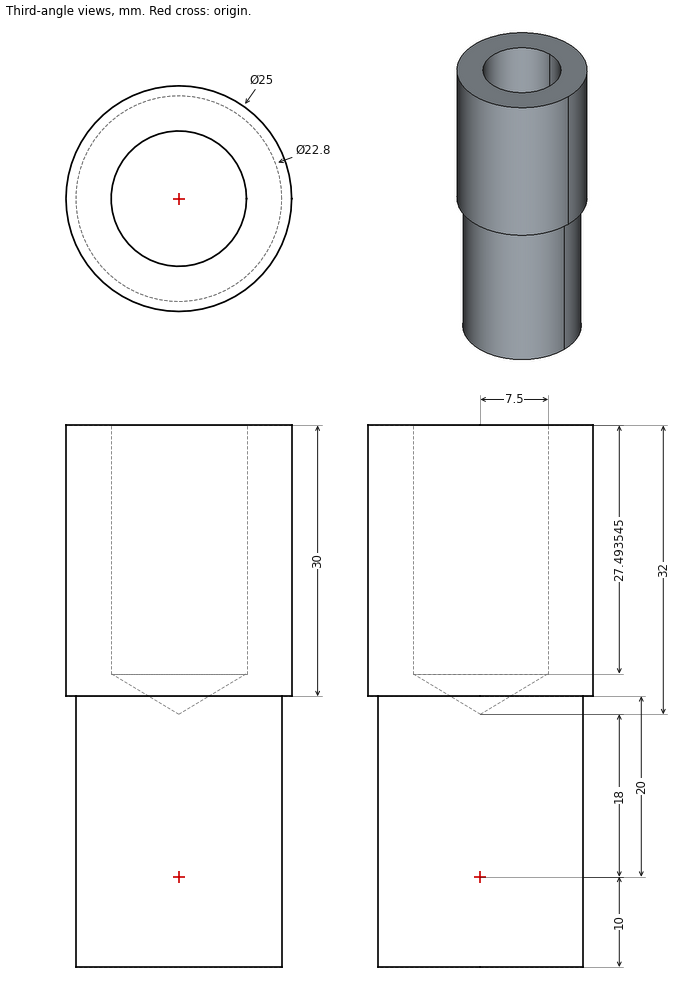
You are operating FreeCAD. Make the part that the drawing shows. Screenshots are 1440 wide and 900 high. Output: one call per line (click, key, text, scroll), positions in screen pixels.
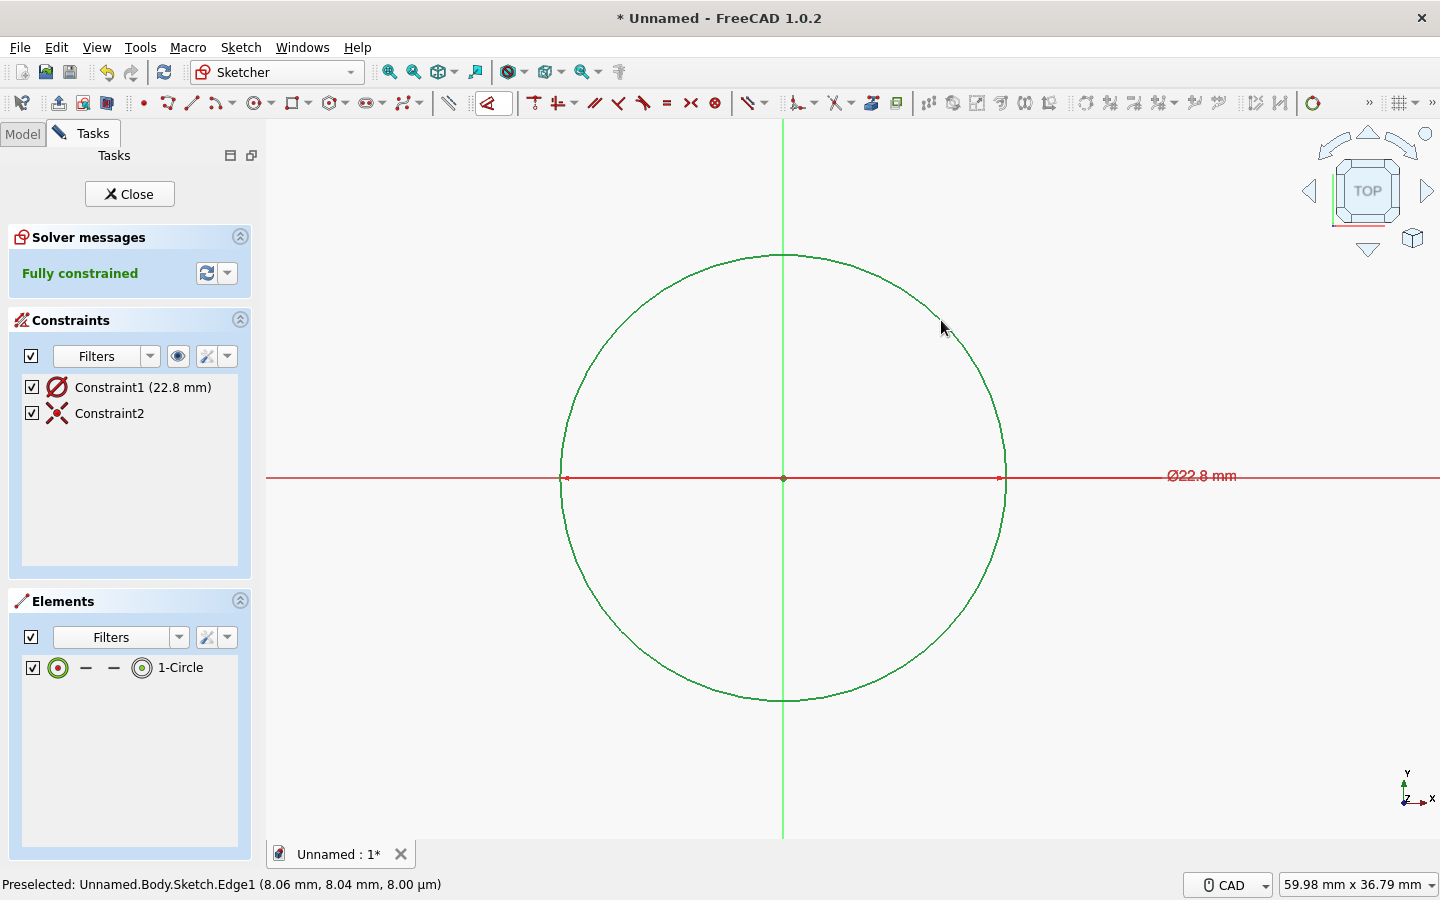
click(130, 194)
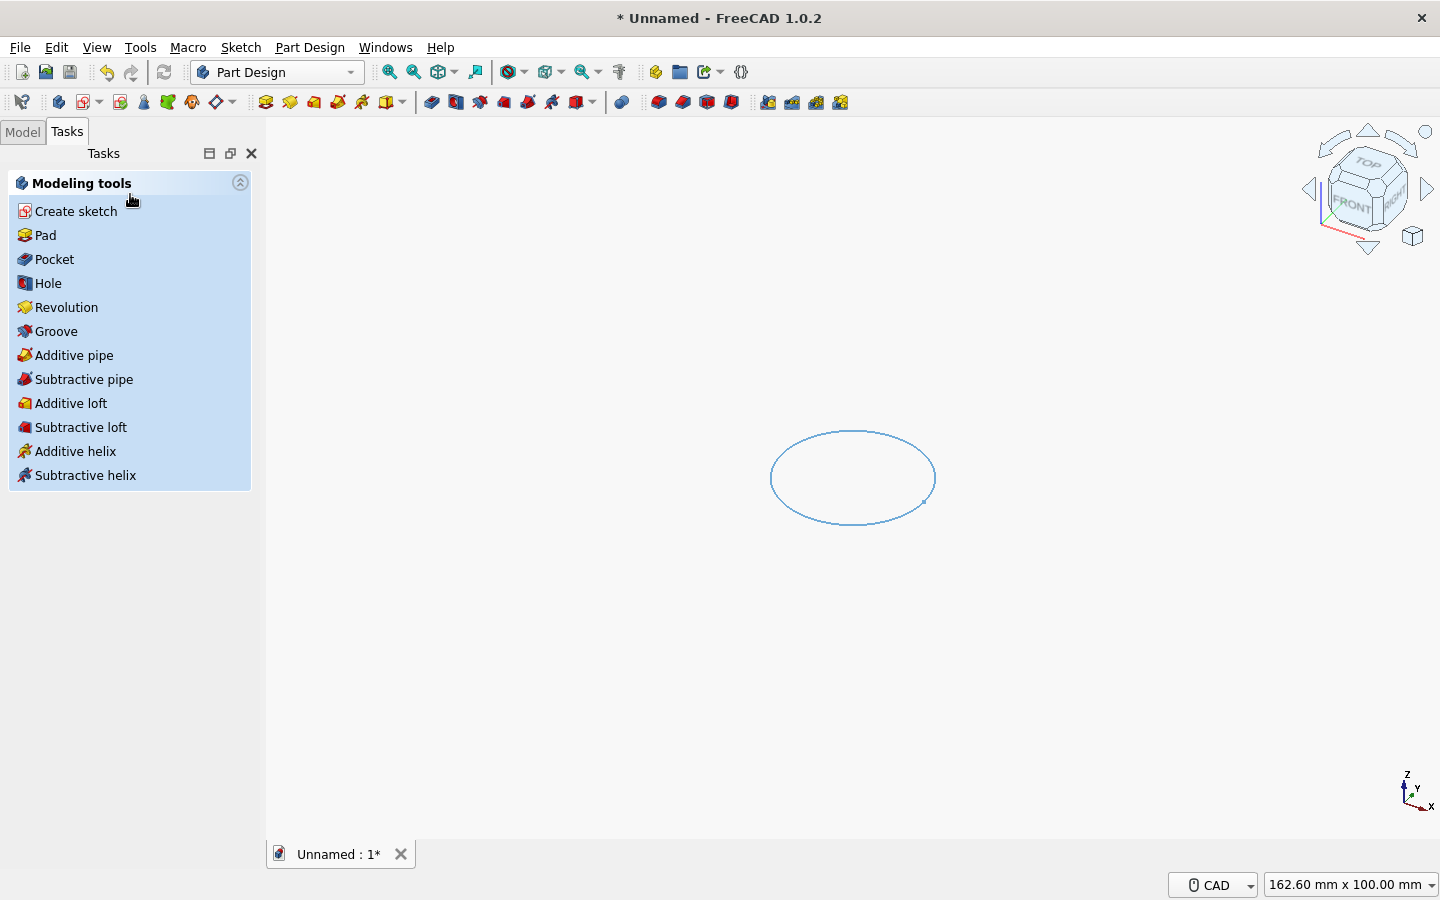
click(266, 102)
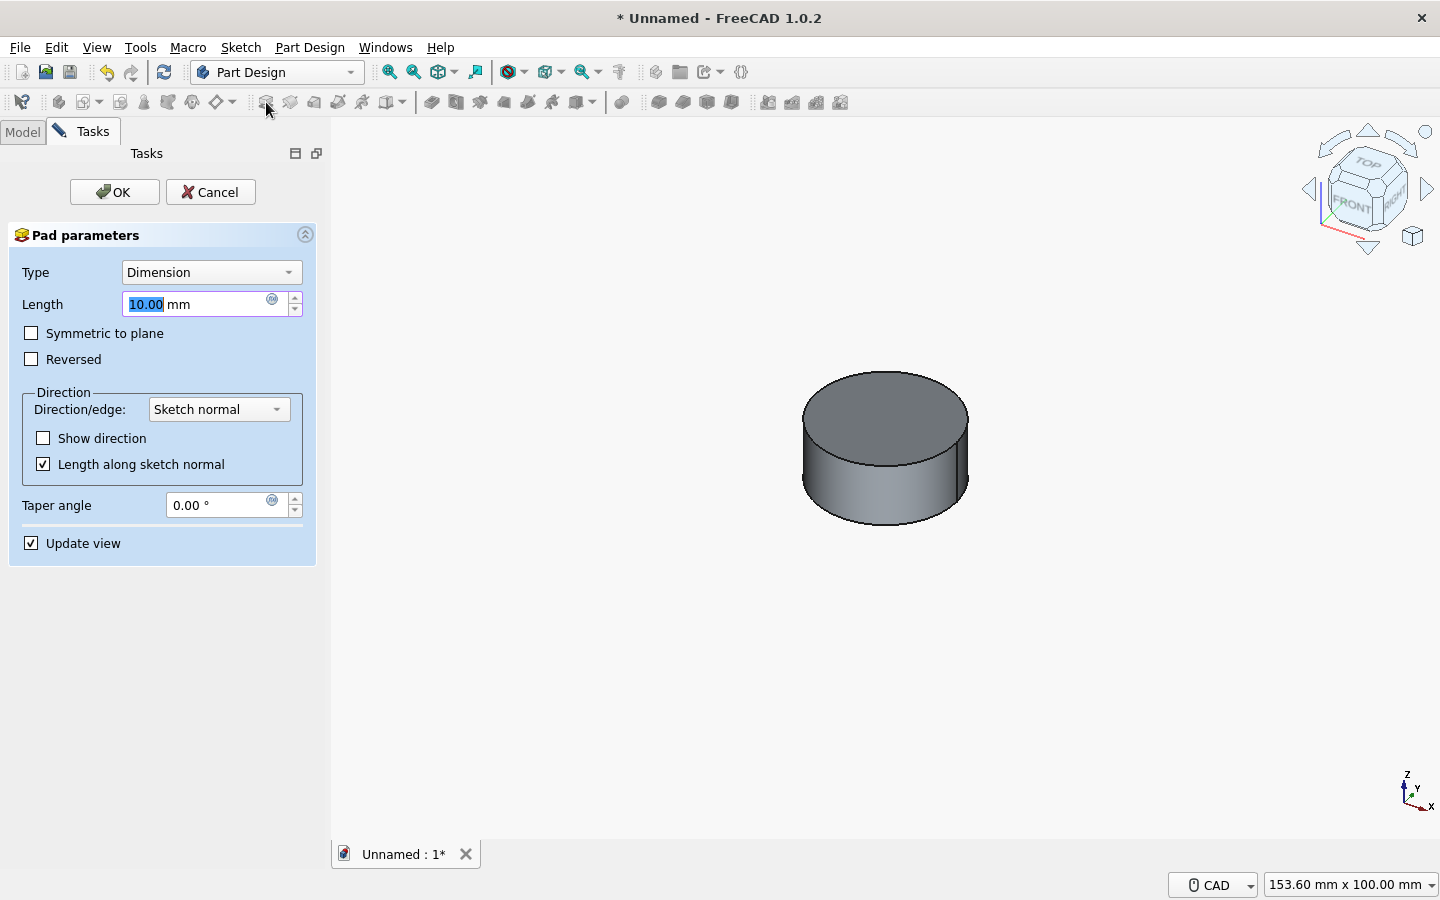
click(212, 272)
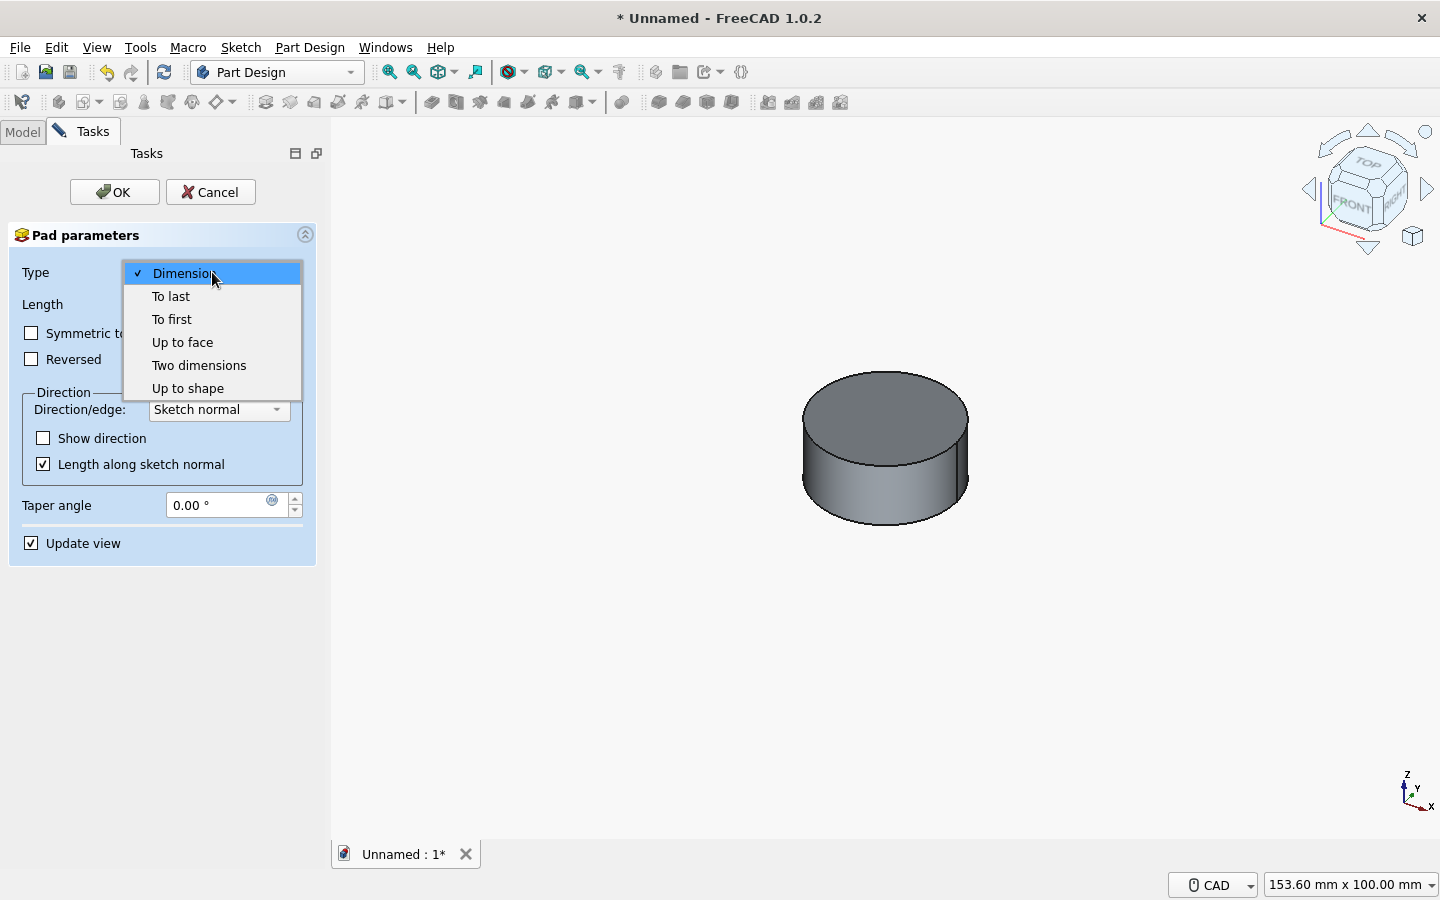
click(212, 366)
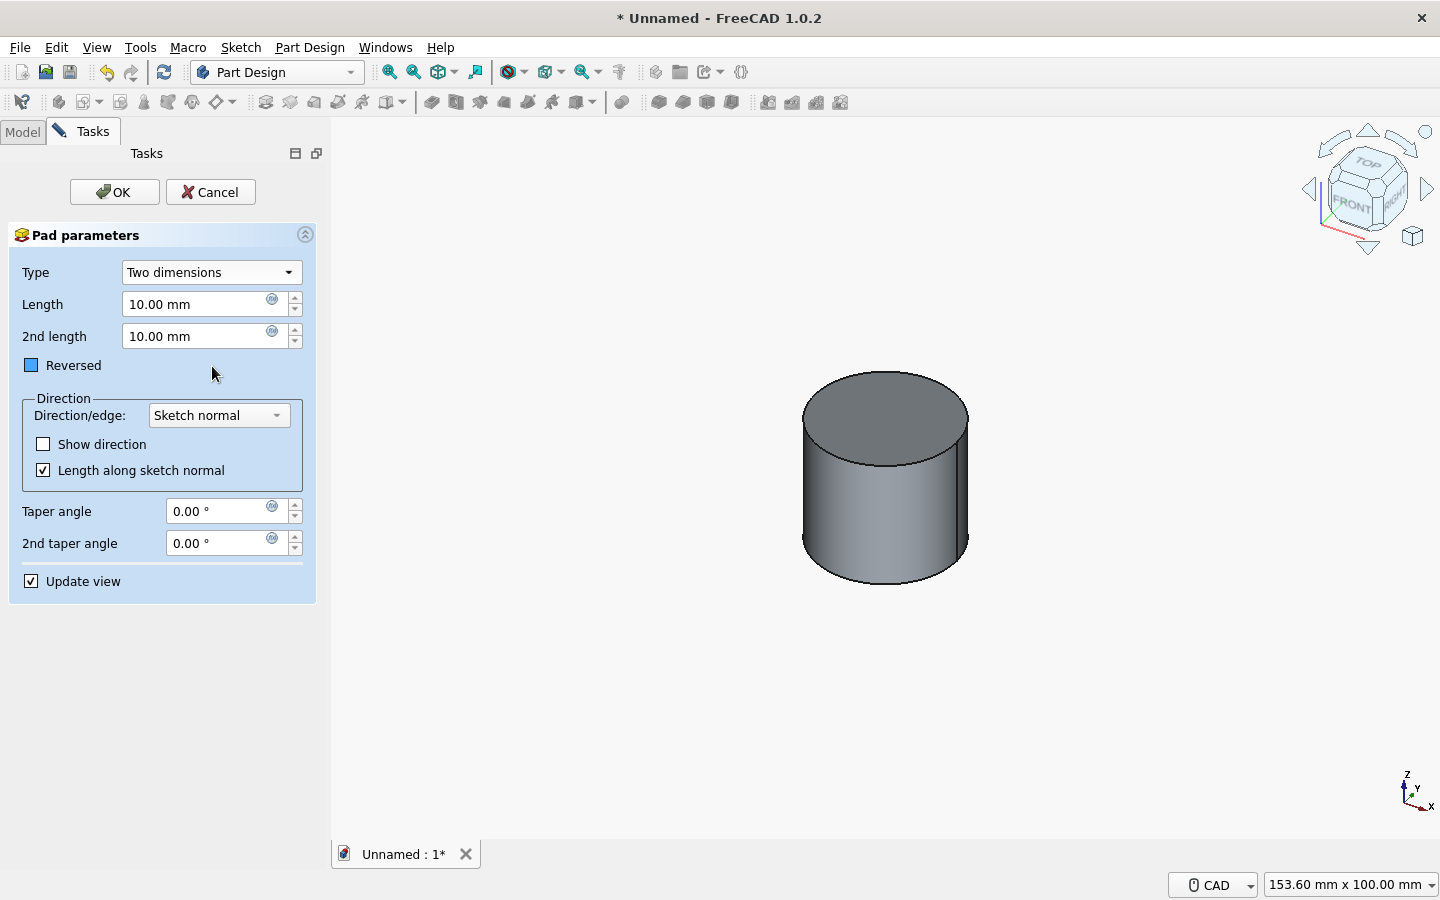
triple_click(204, 304)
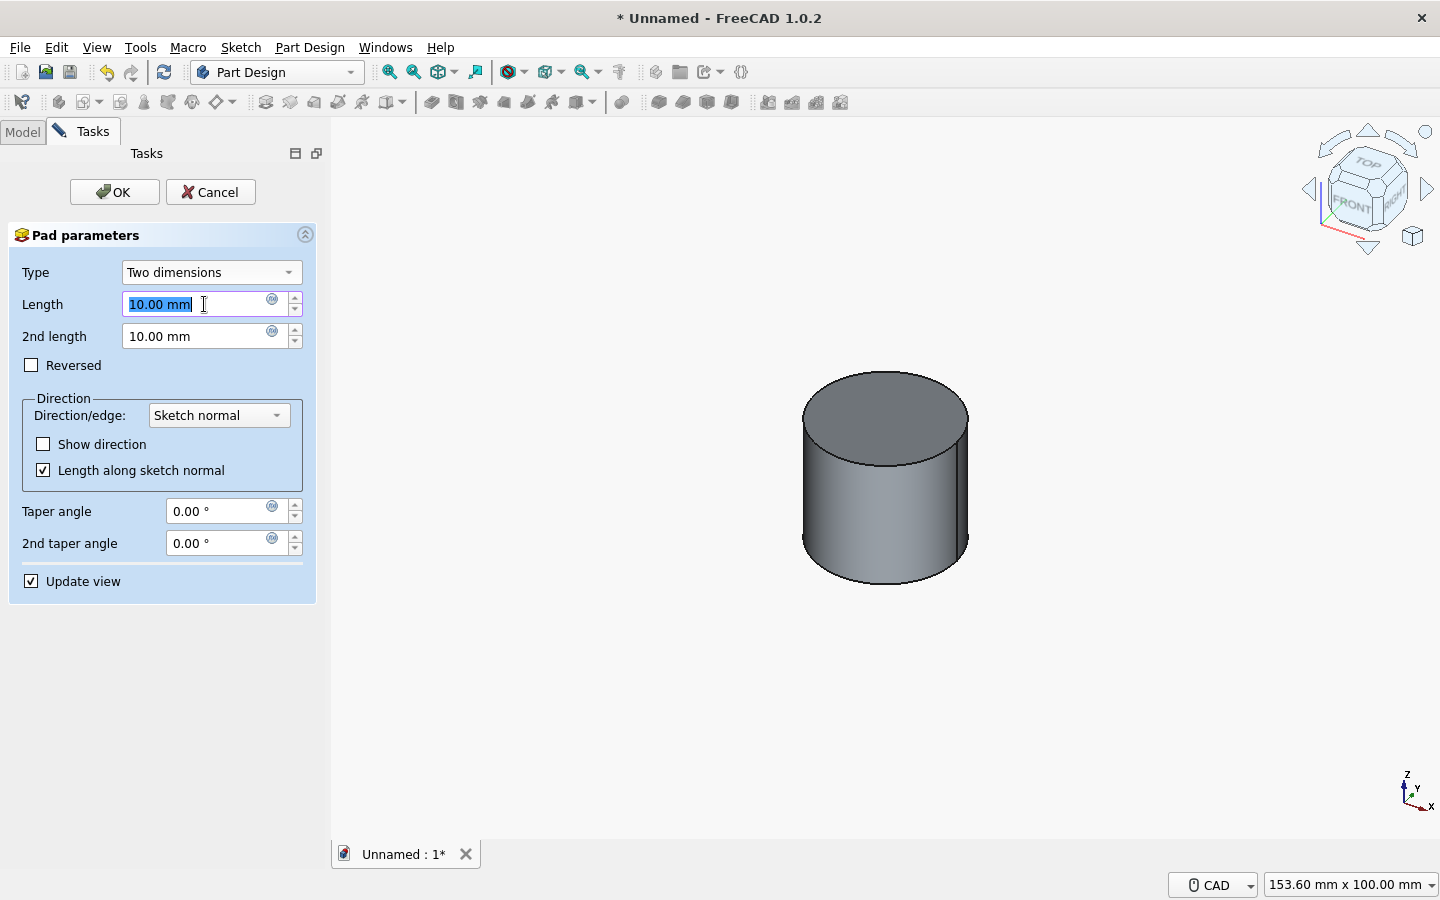
text(20)
key(Tab)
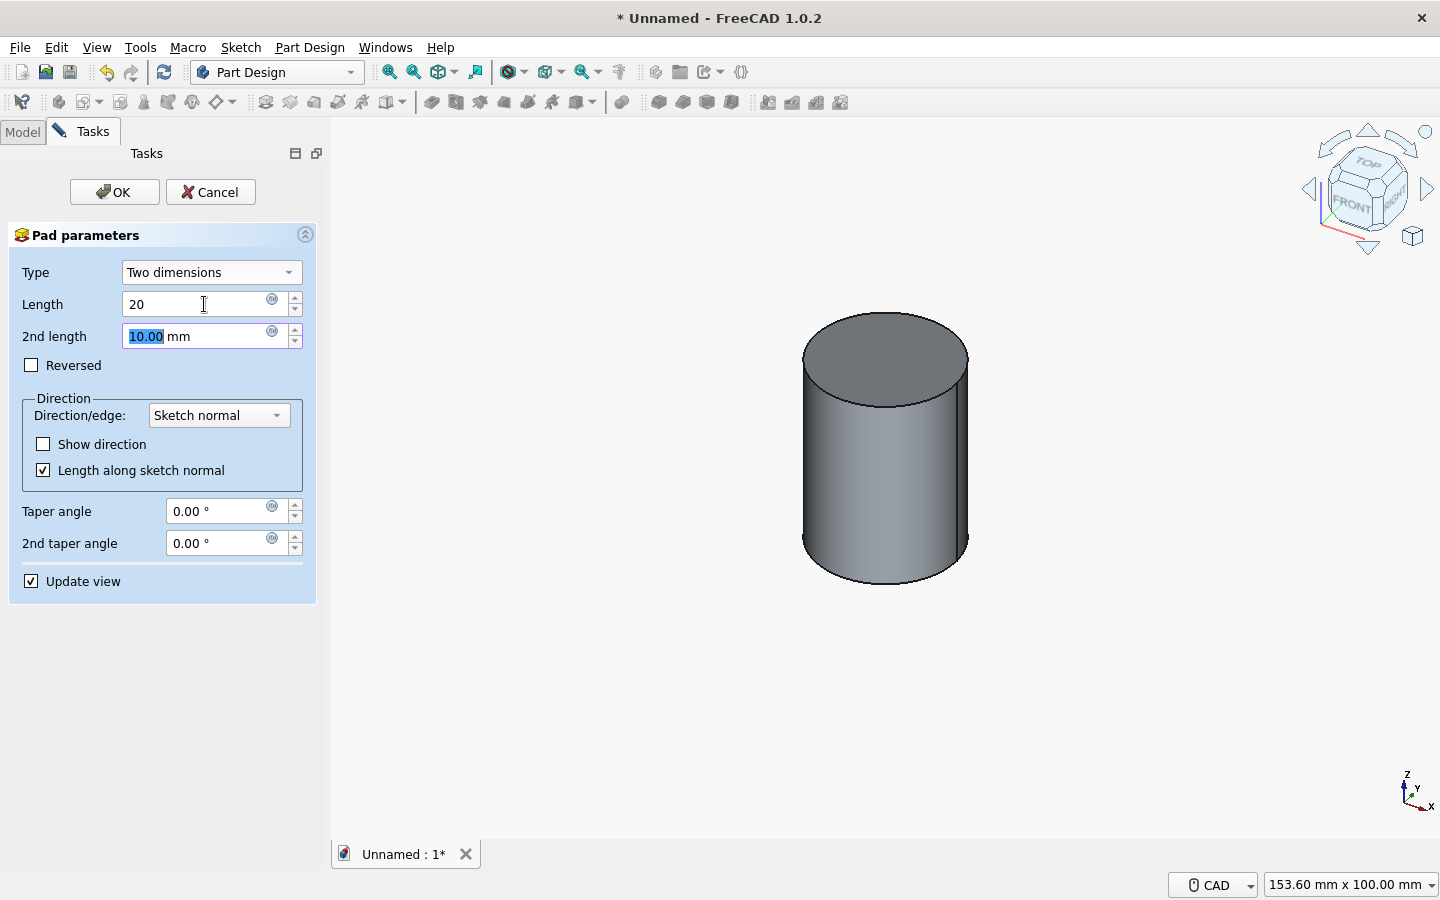
text(10)
key(Tab)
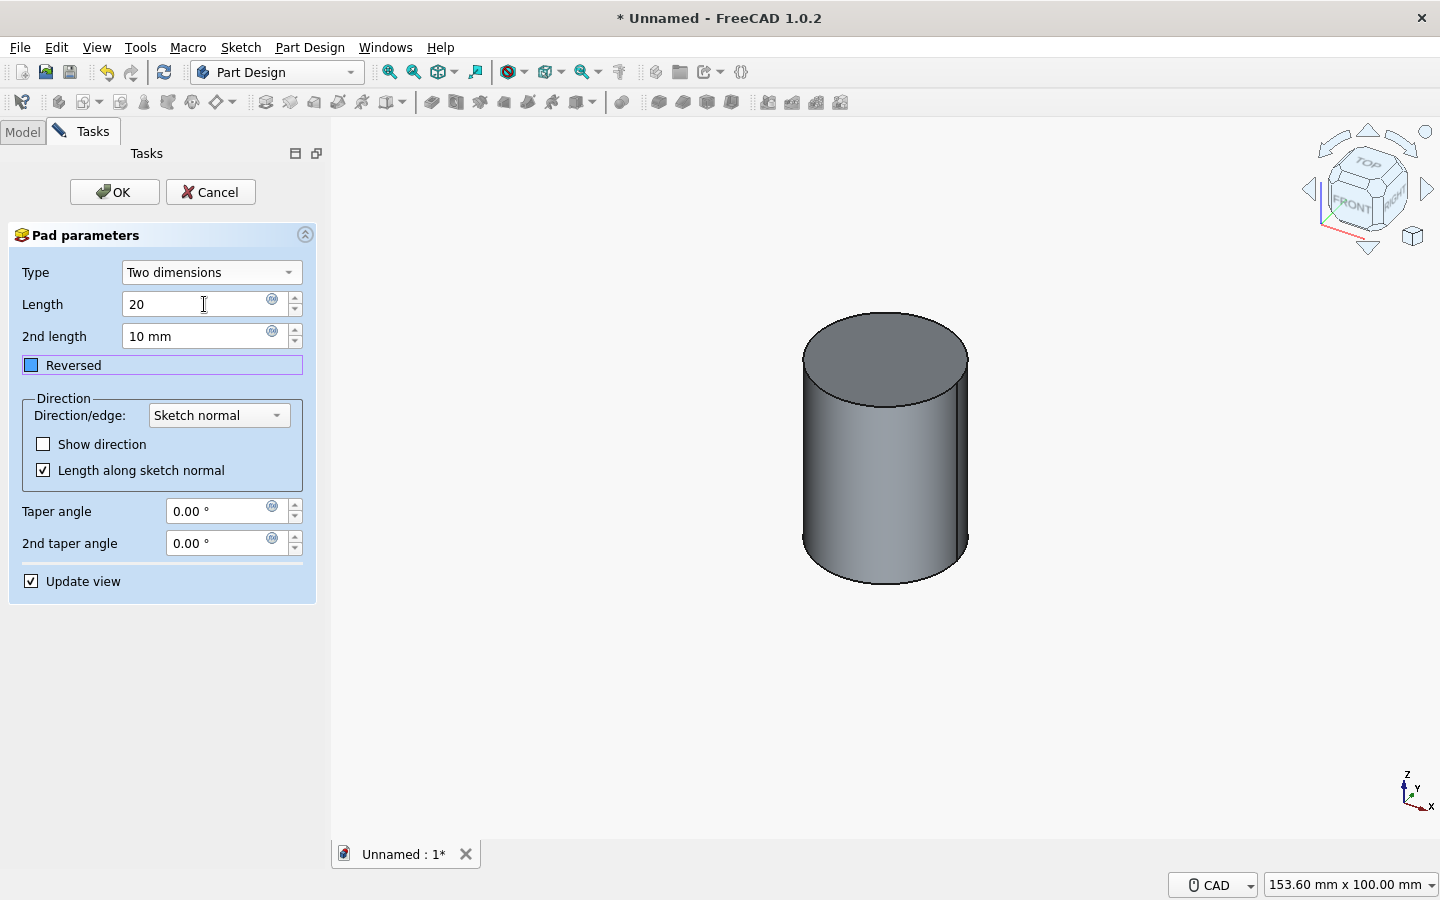
click(115, 192)